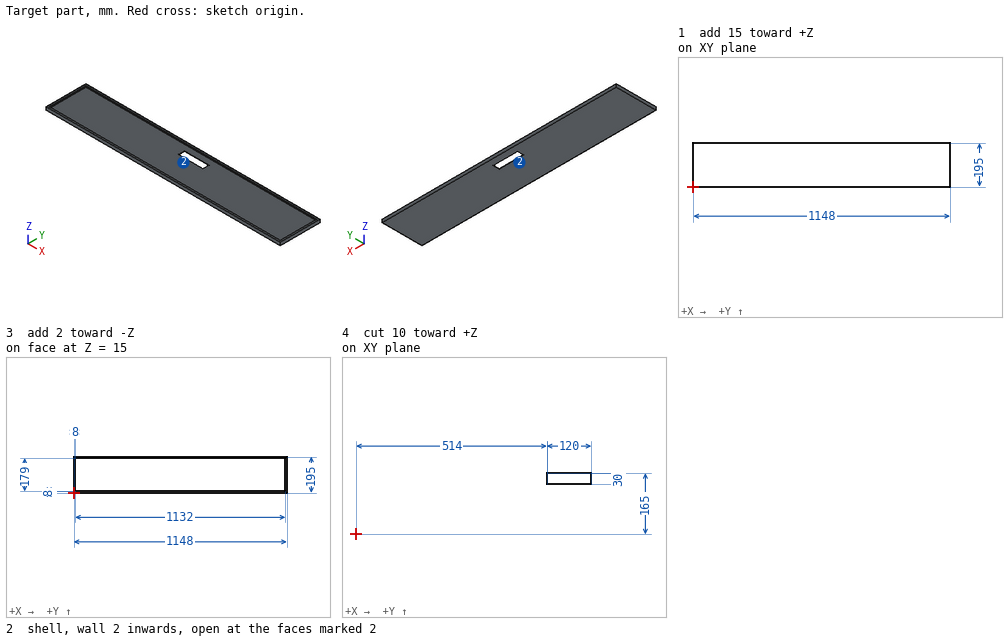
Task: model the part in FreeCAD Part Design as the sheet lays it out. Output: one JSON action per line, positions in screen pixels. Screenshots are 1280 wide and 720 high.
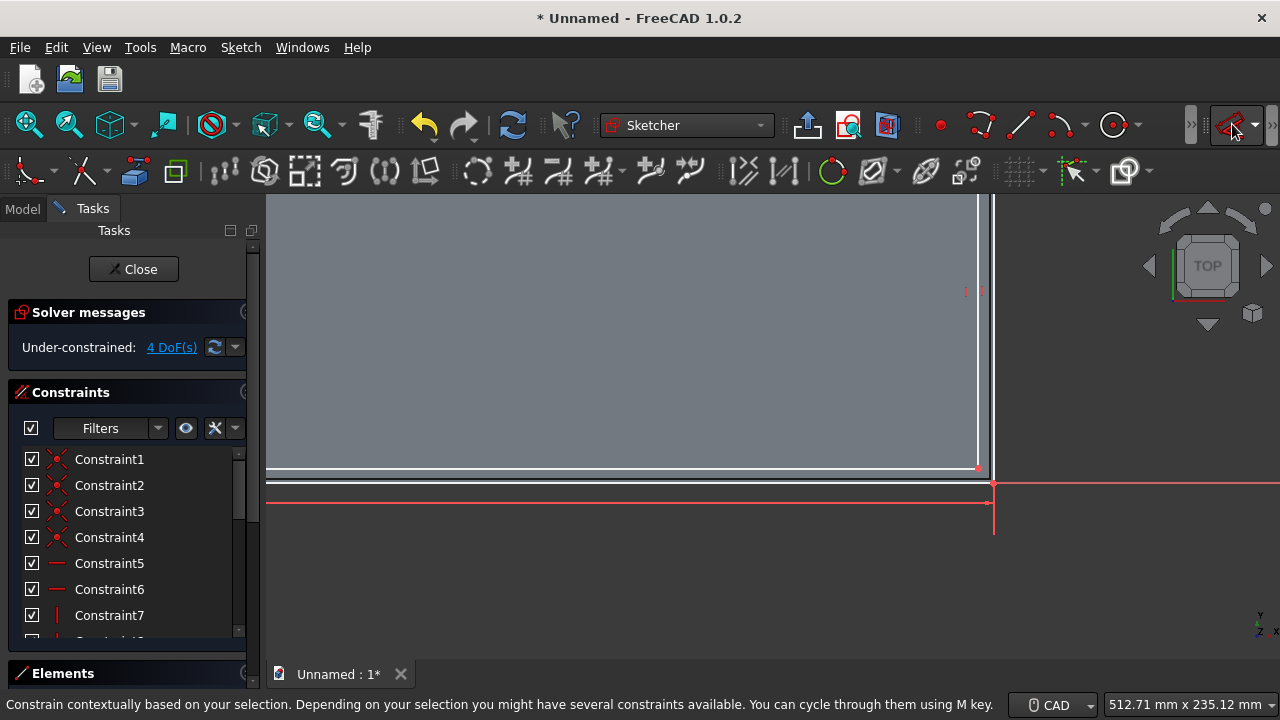
{"action": "scroll", "coordinate": [981, 471], "scroll_direction": "down", "scroll_amount": 7}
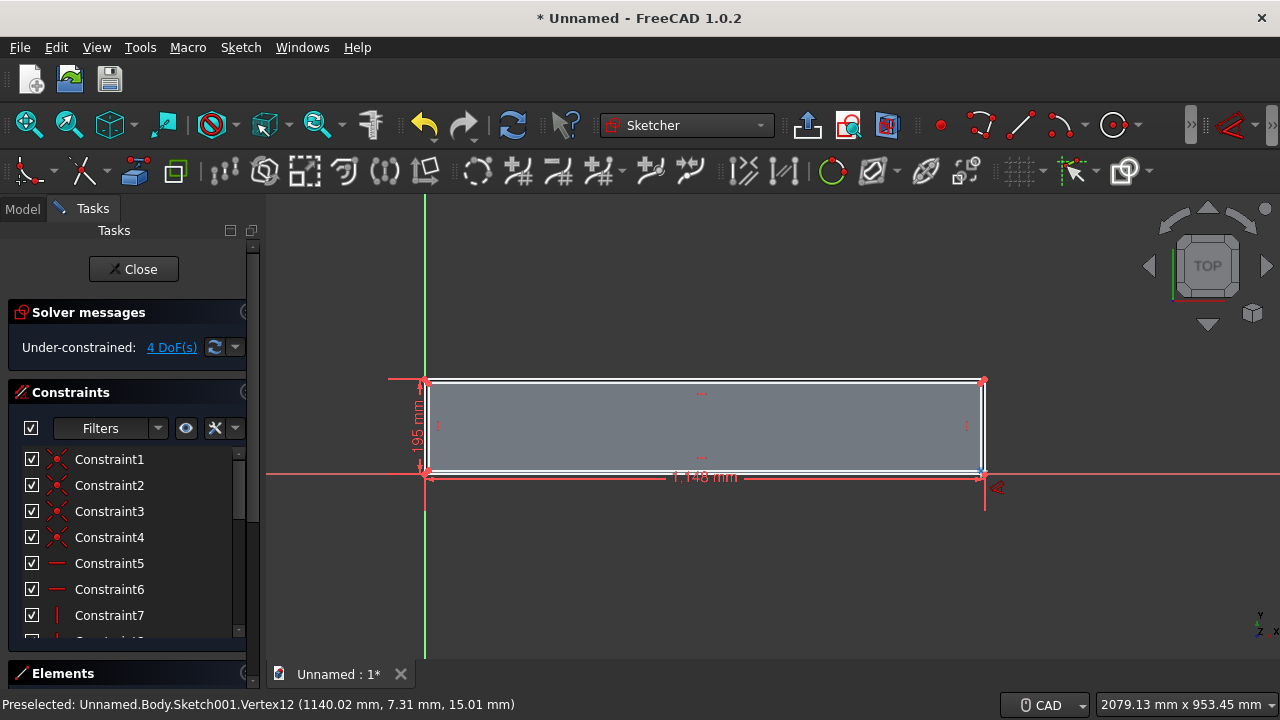
{"action": "scroll", "coordinate": [429, 383], "scroll_direction": "up", "scroll_amount": 12}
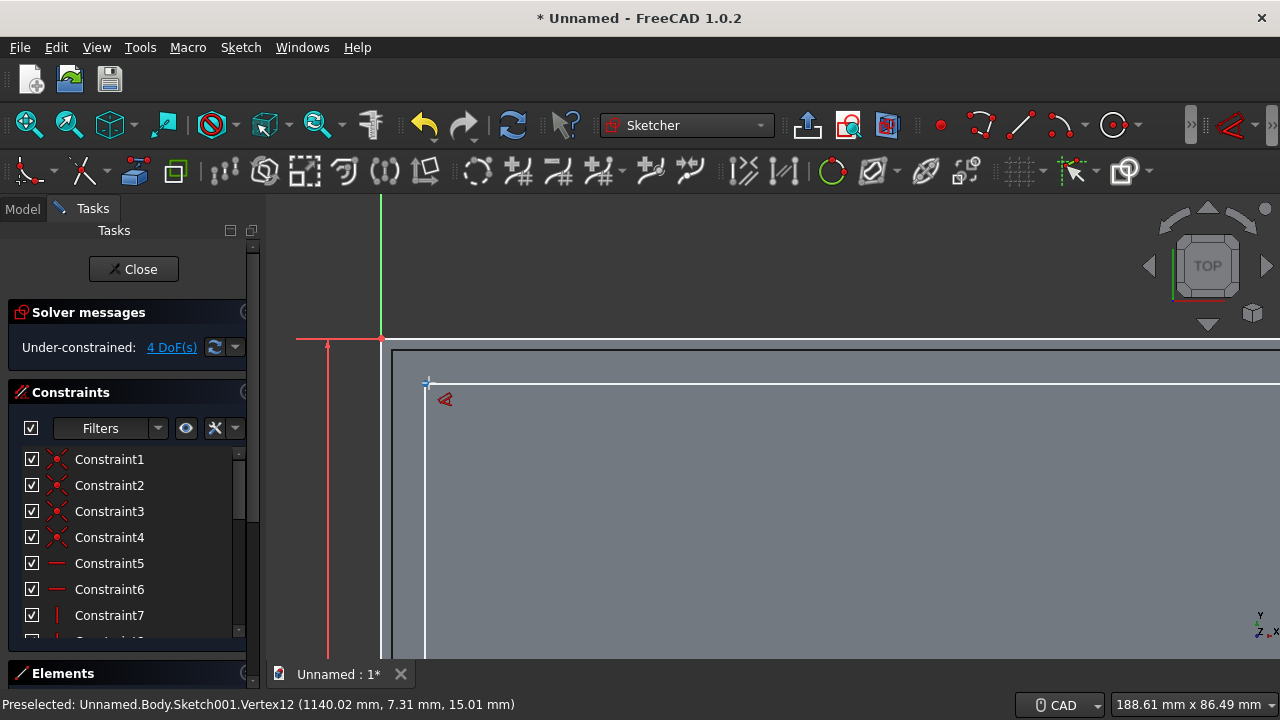
{"action": "left_click", "coordinate": [425, 384]}
{"action": "left_click", "coordinate": [403, 326]}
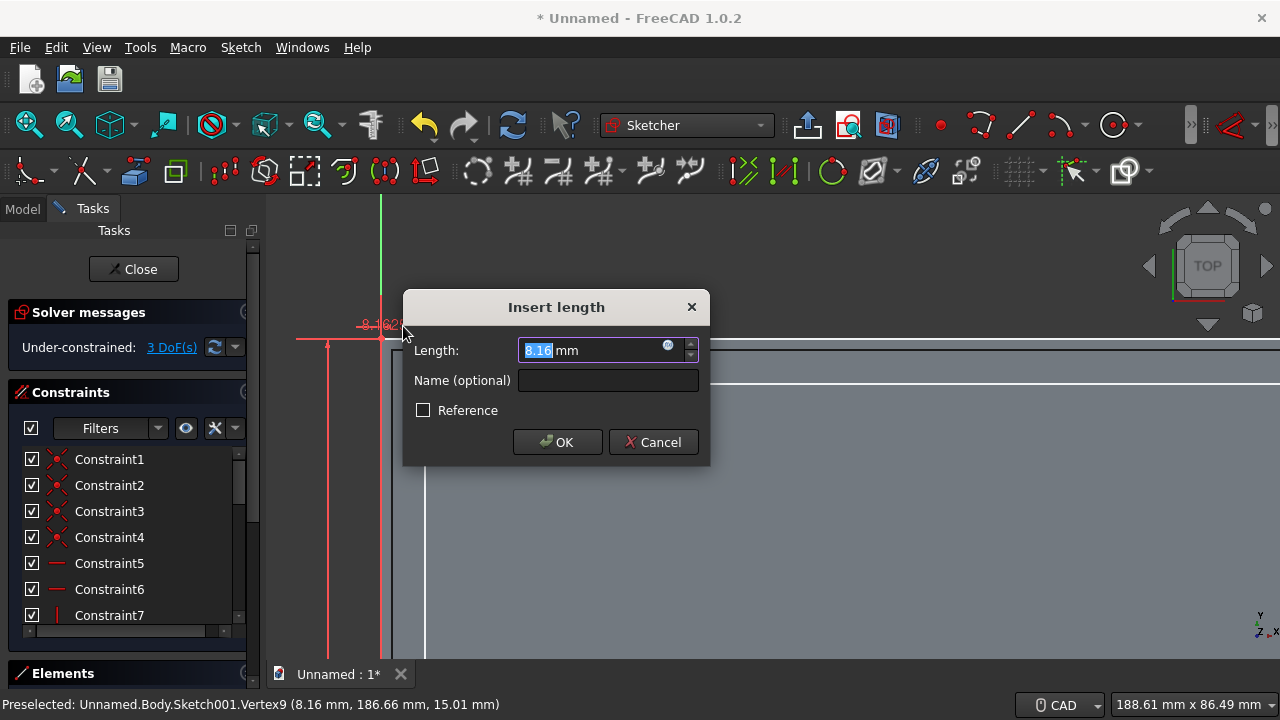
{"action": "type", "text": "8"}
{"action": "key", "text": "Return"}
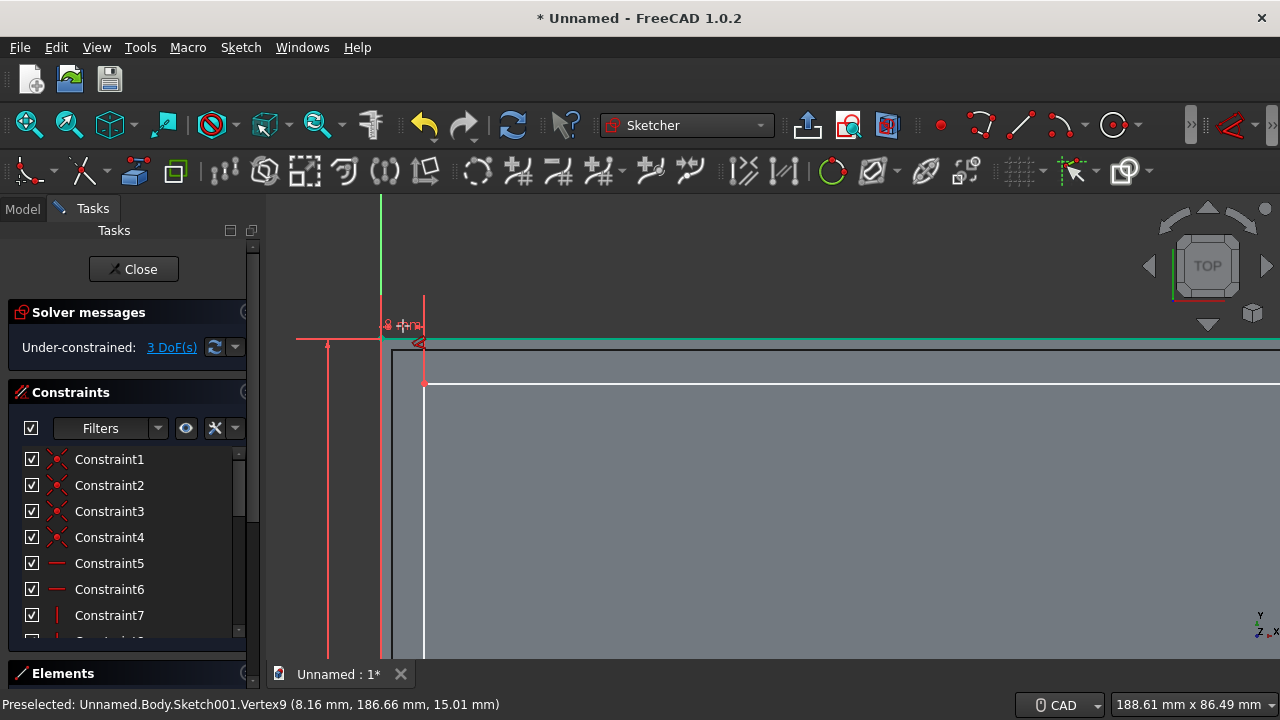
{"action": "scroll", "coordinate": [429, 383], "scroll_direction": "down", "scroll_amount": 12}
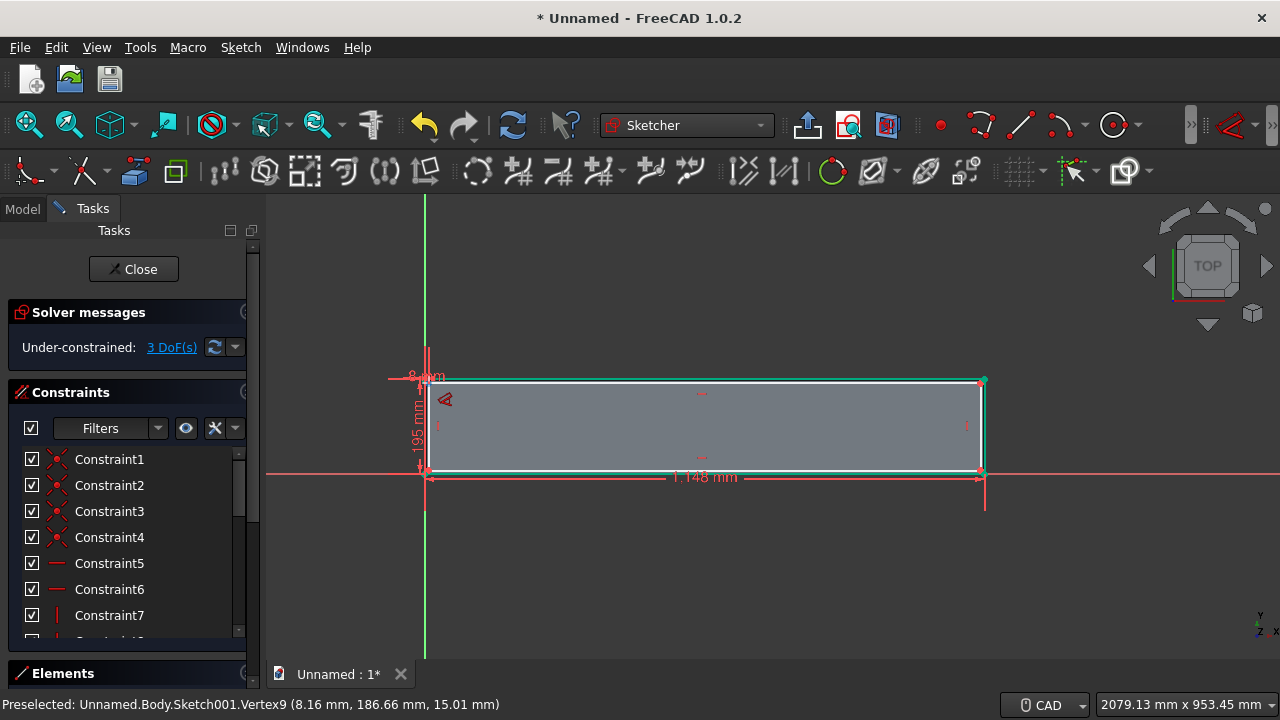
{"action": "scroll", "coordinate": [429, 471], "scroll_direction": "up", "scroll_amount": 12}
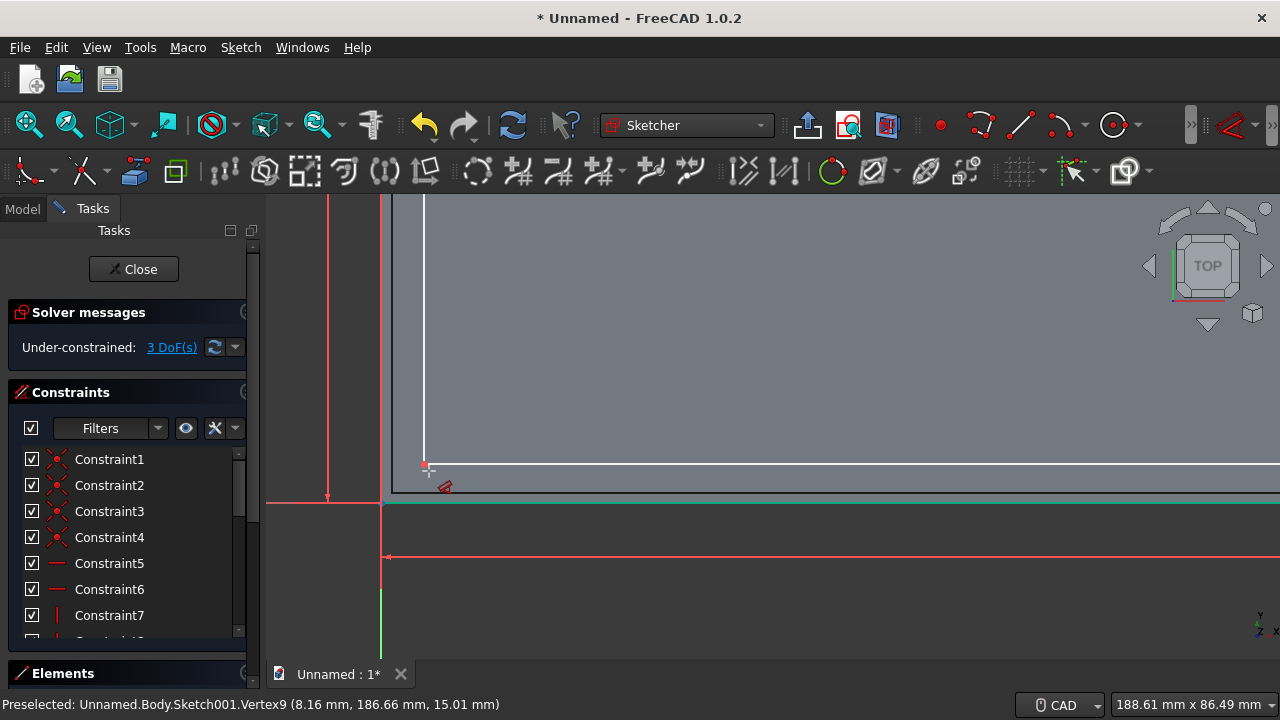
{"action": "left_click", "coordinate": [424, 464]}
{"action": "left_click", "coordinate": [347, 484]}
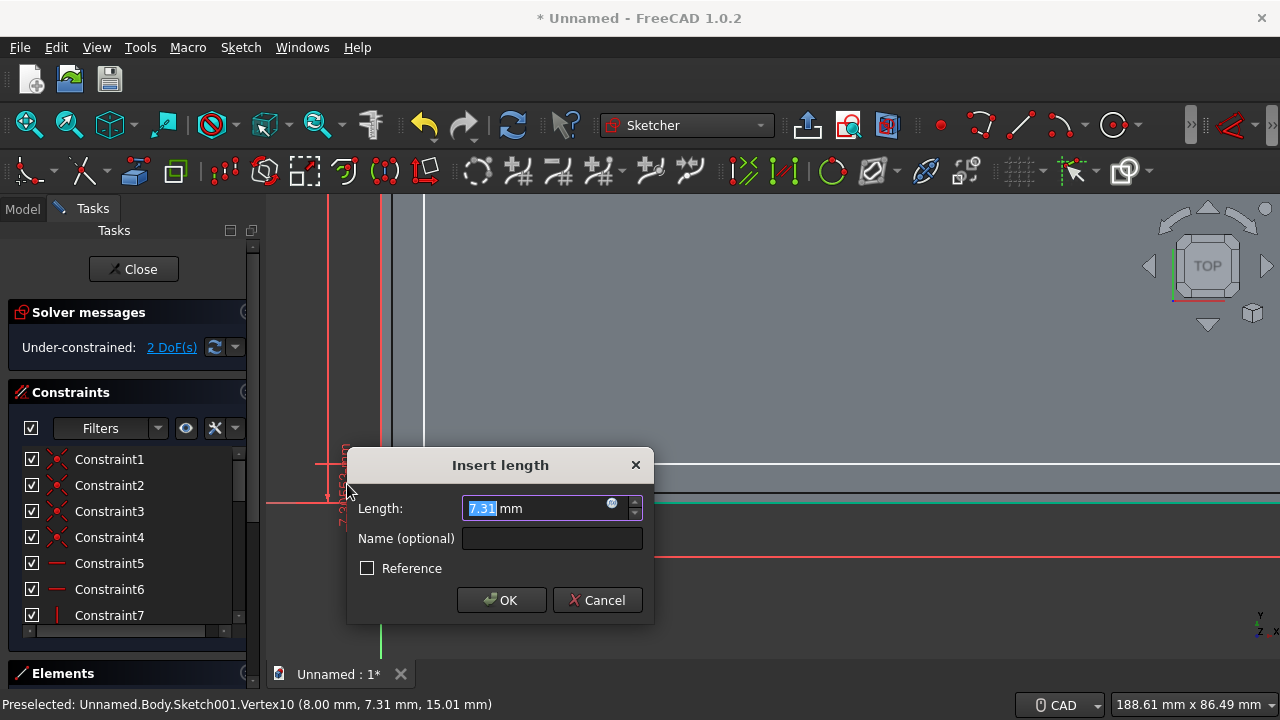
{"action": "type", "text": "8"}
{"action": "key", "text": "Return"}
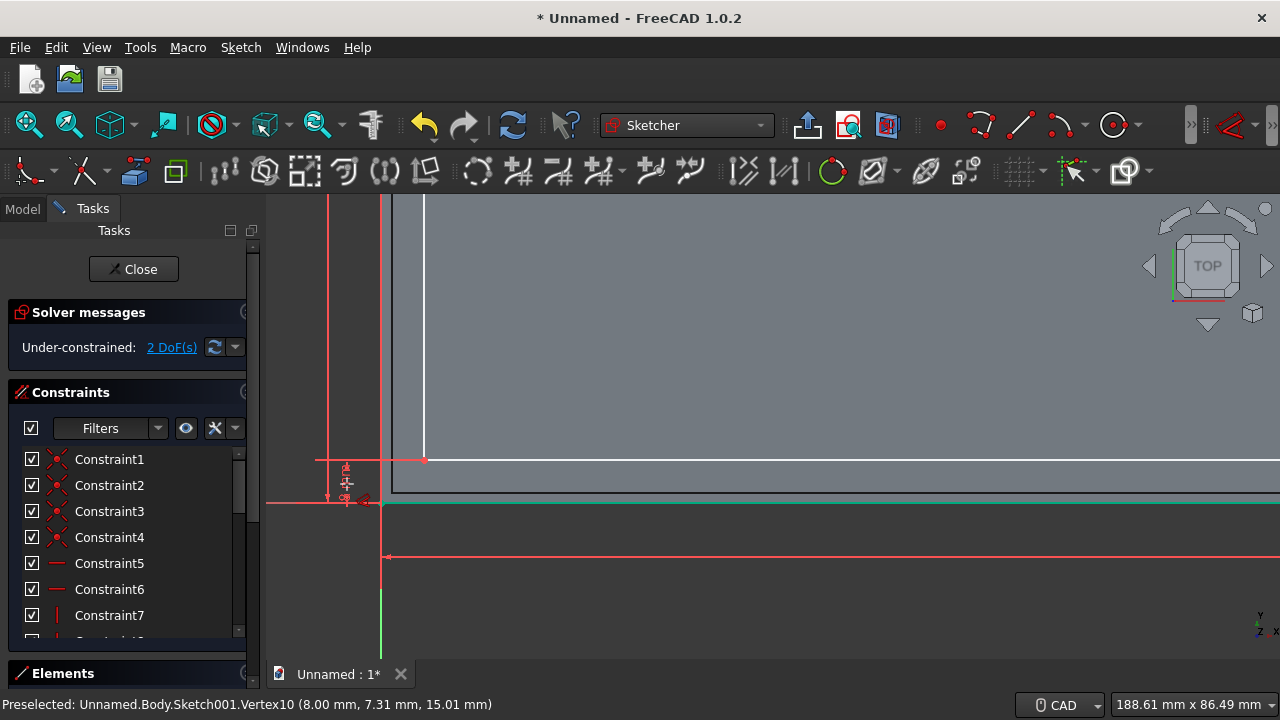
{"action": "scroll", "coordinate": [429, 471], "scroll_direction": "down", "scroll_amount": 12}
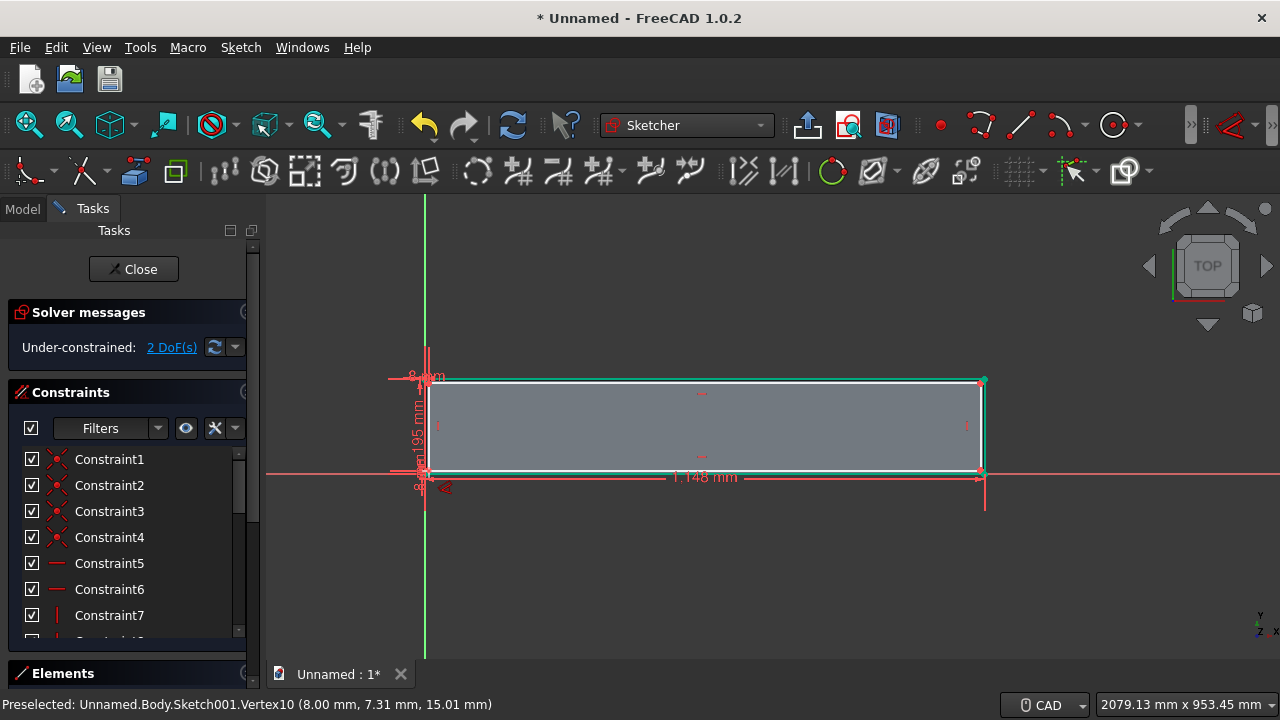
{"action": "scroll", "coordinate": [429, 453], "scroll_direction": "up", "scroll_amount": 7}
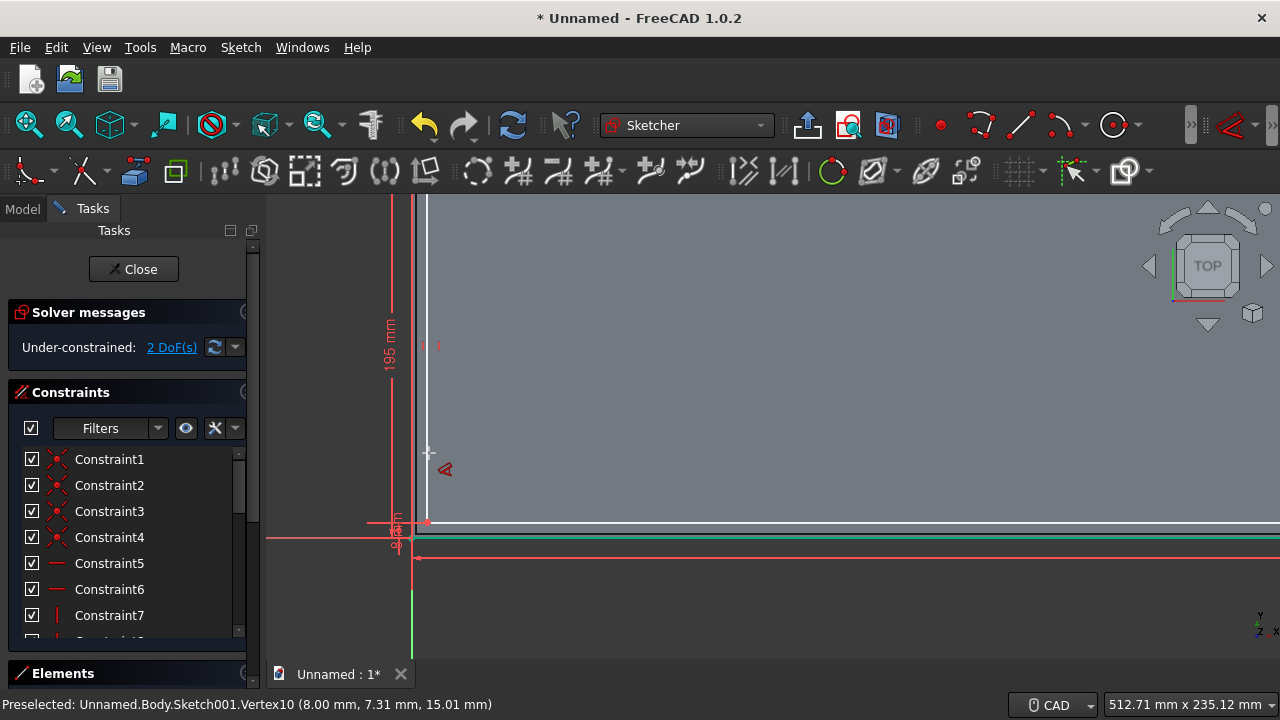
{"action": "left_click", "coordinate": [427, 452]}
{"action": "left_click", "coordinate": [393, 372]}